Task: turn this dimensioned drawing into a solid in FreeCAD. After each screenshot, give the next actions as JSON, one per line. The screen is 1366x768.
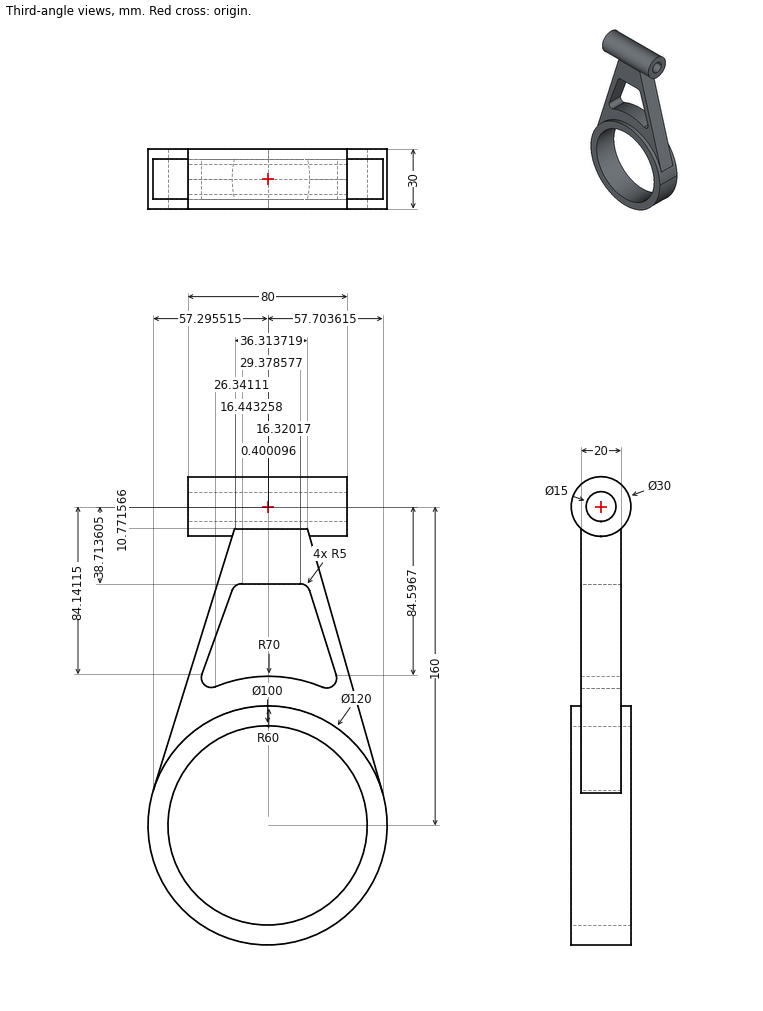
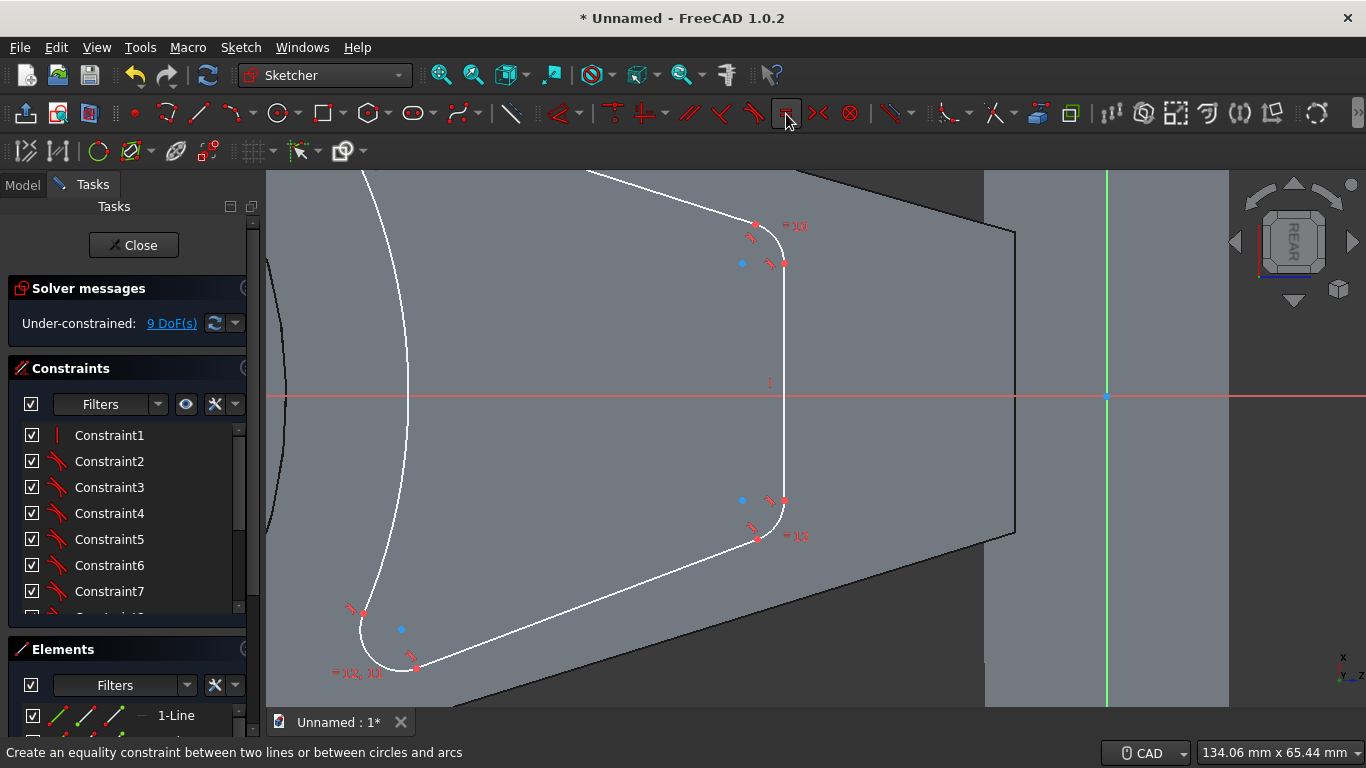
{"action": "left_click", "coordinate": [558, 114]}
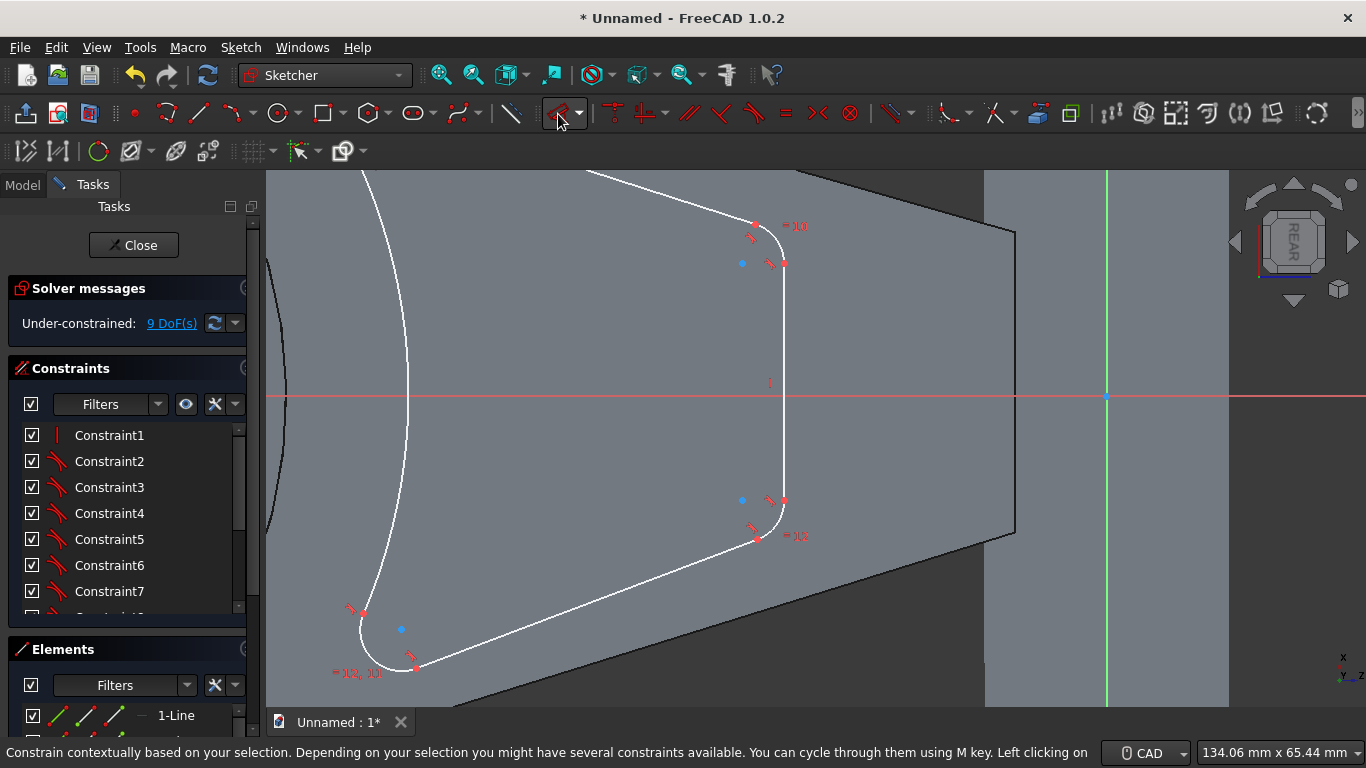
{"action": "left_click", "coordinate": [781, 248]}
{"action": "left_click", "coordinate": [811, 236]}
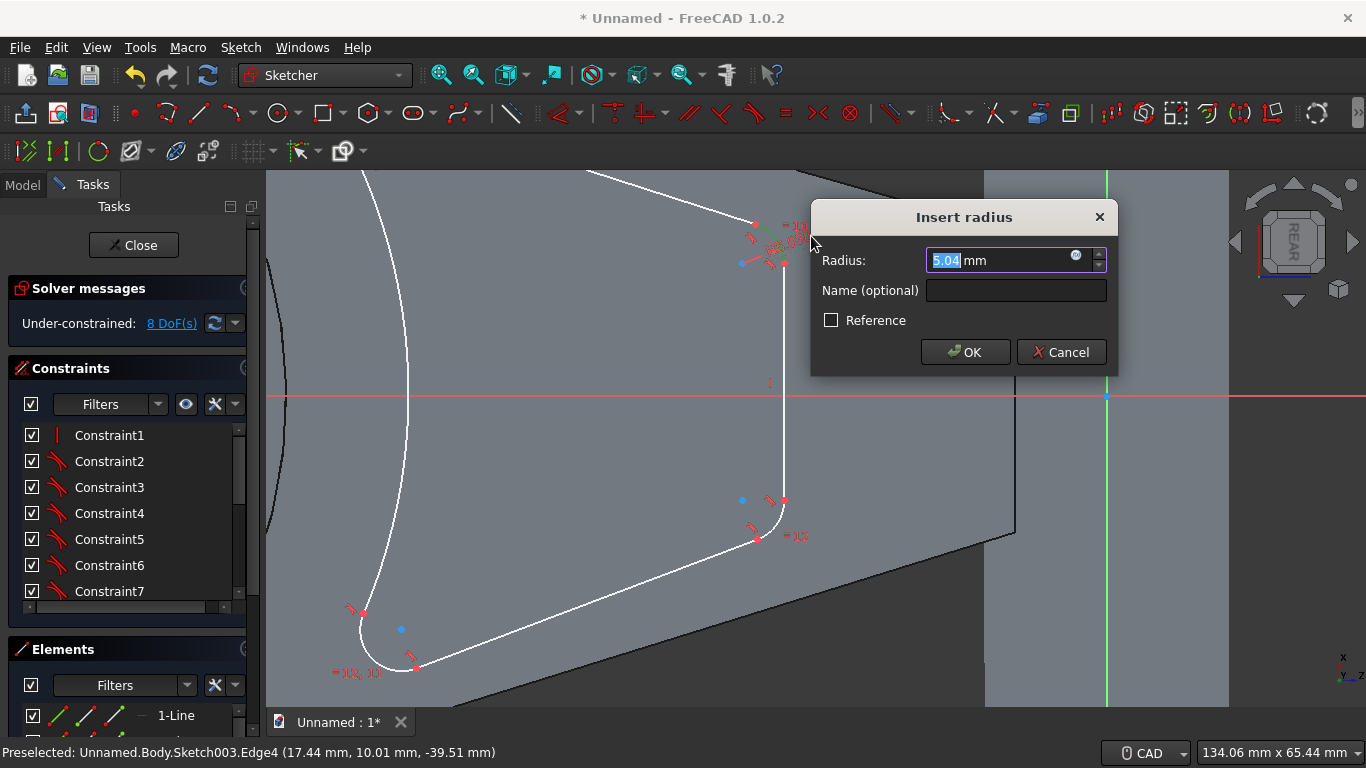
{"action": "type", "text": "5"}
{"action": "key", "text": "Return"}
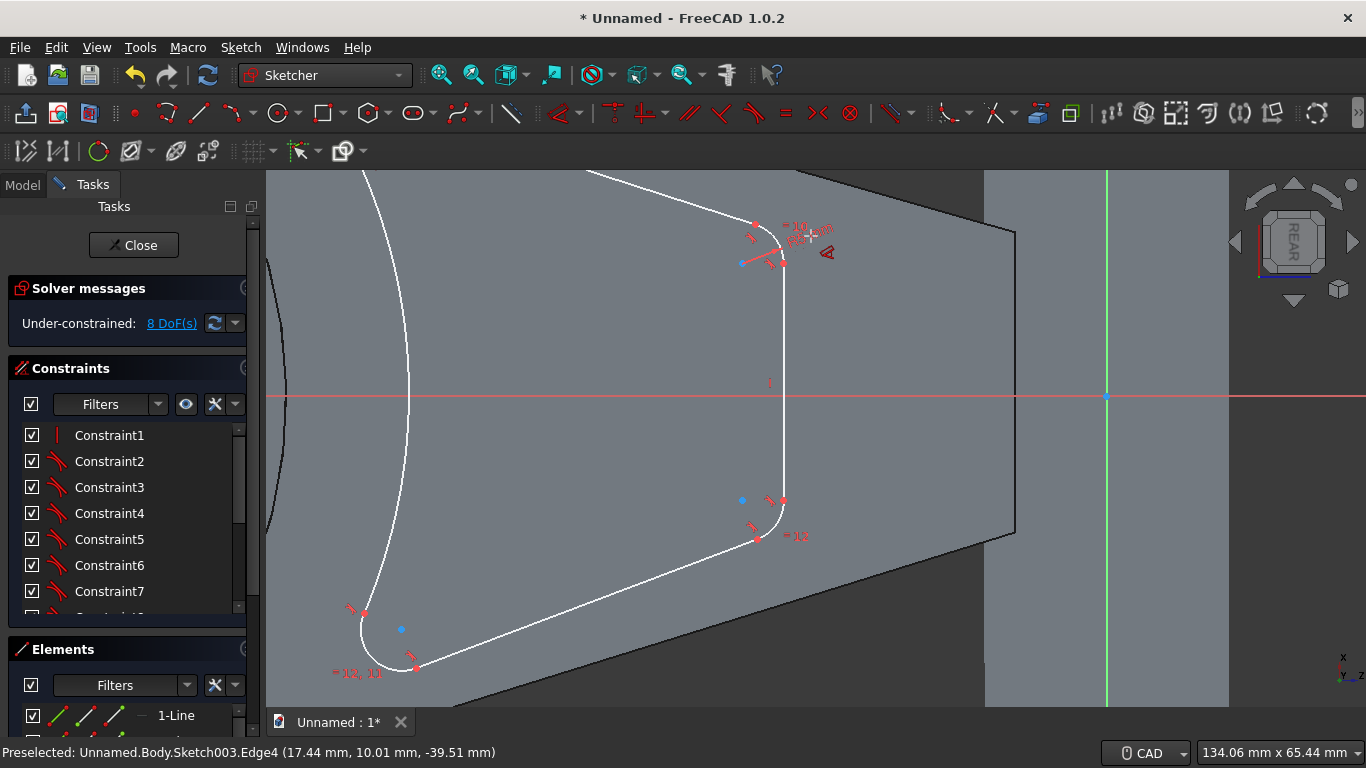
{"action": "left_click", "coordinate": [402, 482]}
{"action": "left_click", "coordinate": [434, 487]}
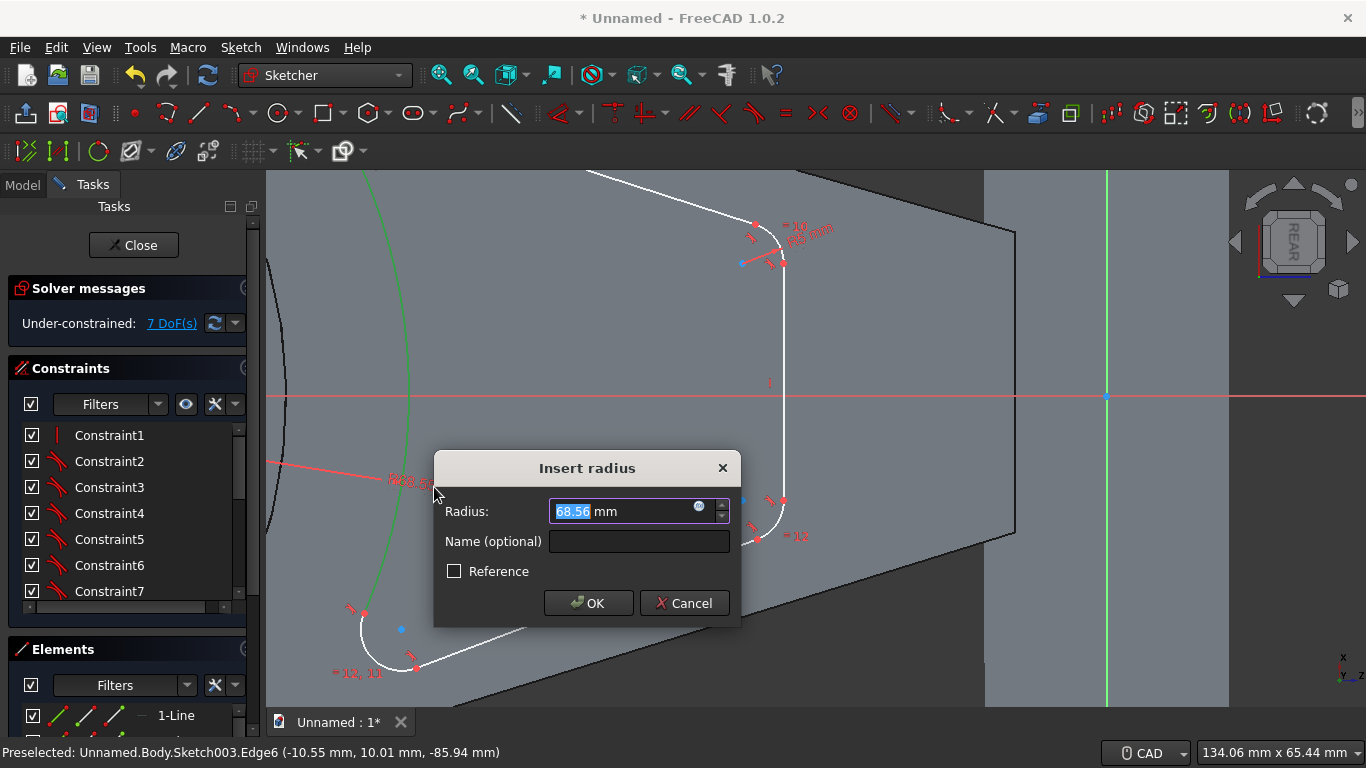
{"action": "type", "text": "70"}
{"action": "key", "text": "Return"}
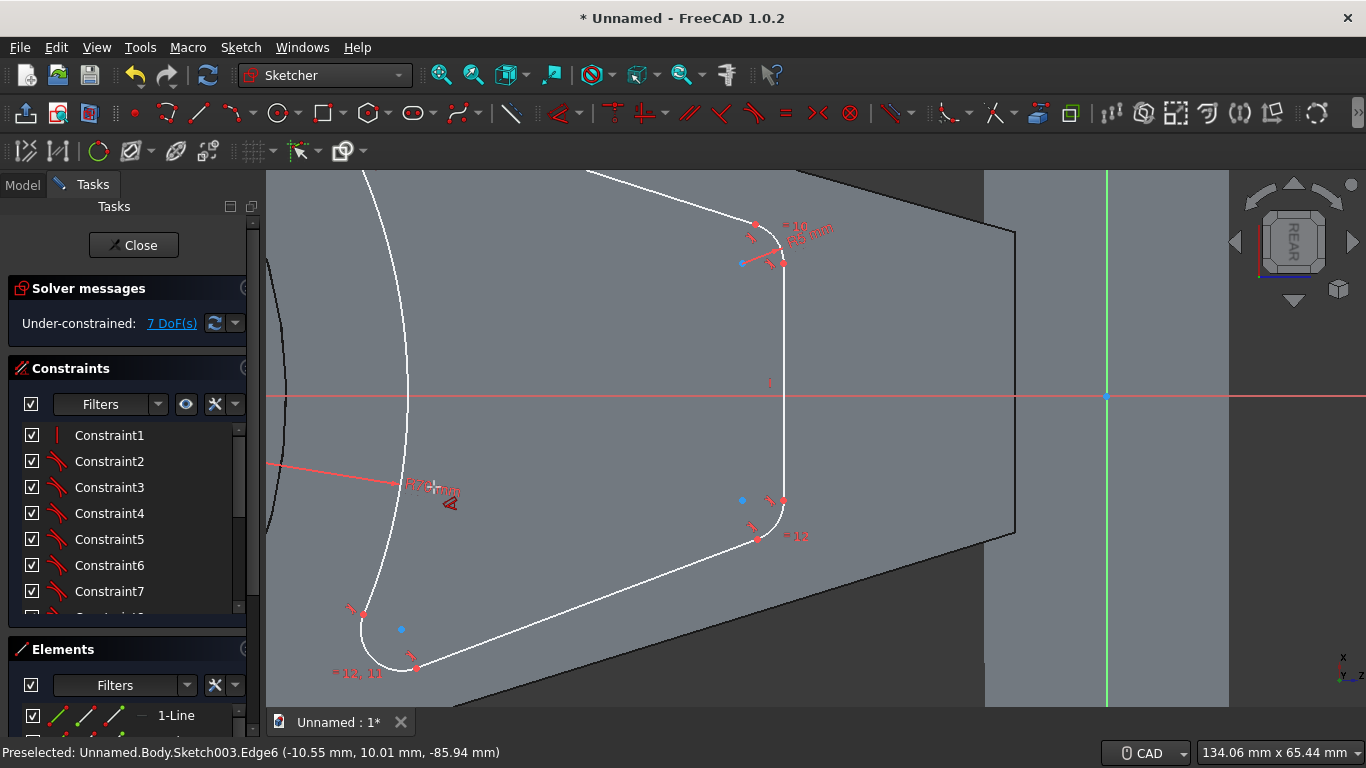
{"action": "scroll", "coordinate": [773, 537], "scroll_direction": "down", "scroll_amount": 2}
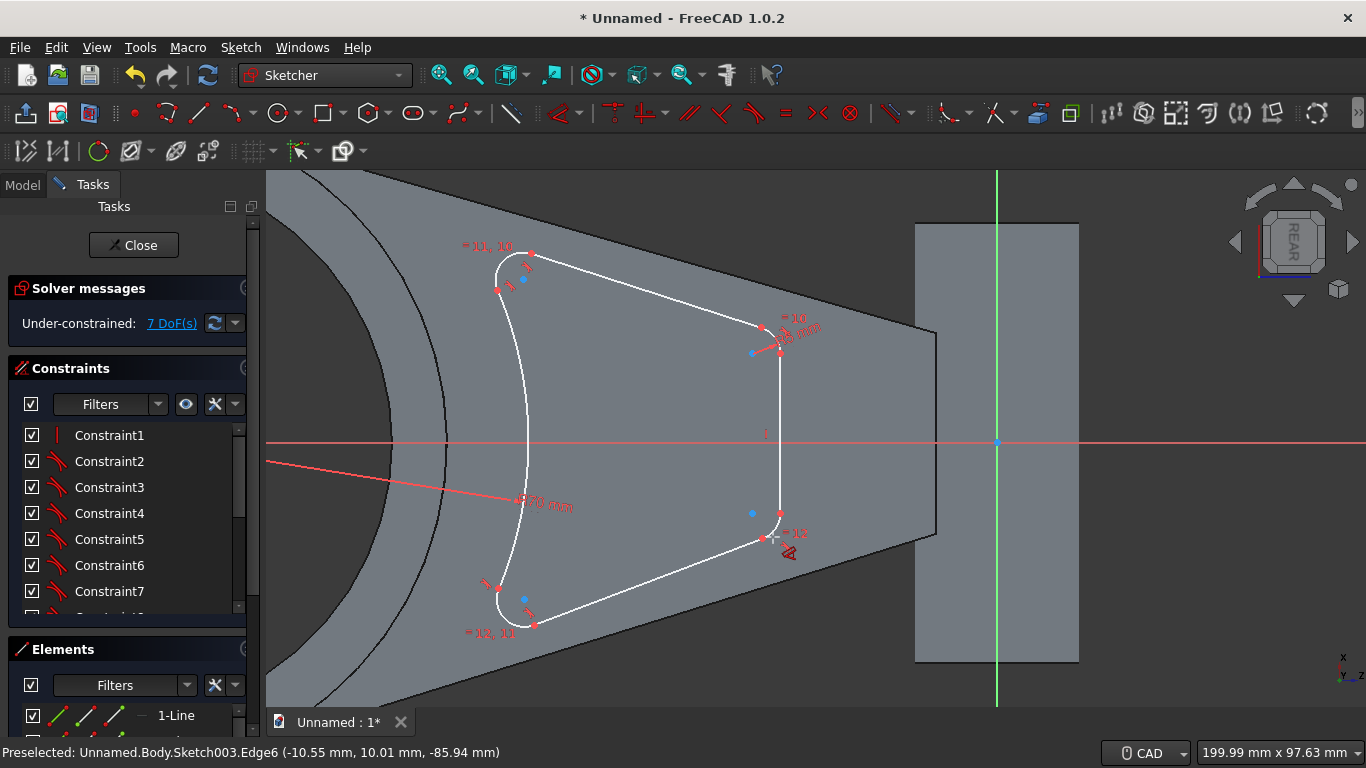
{"action": "left_click", "coordinate": [532, 254]}
{"action": "left_click", "coordinate": [764, 220]}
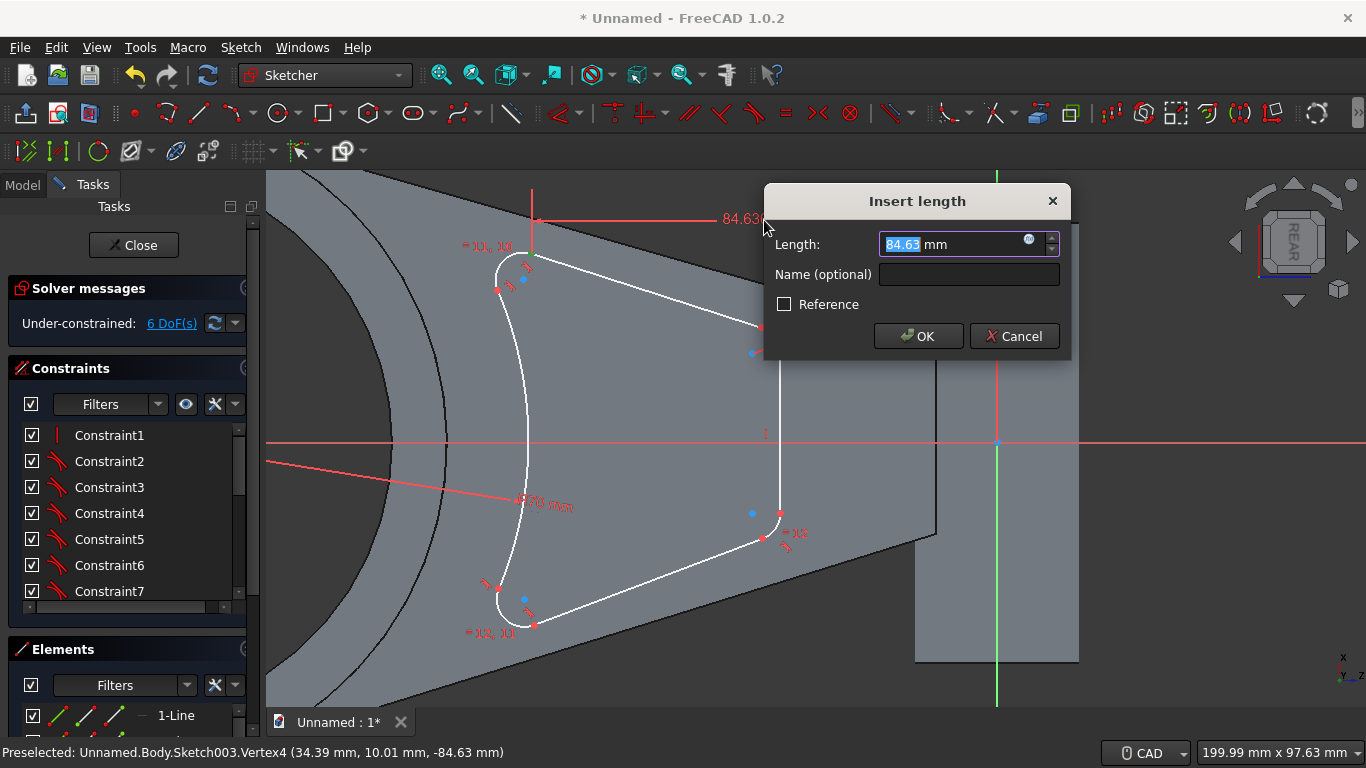
{"action": "type", "text": "84.5967"}
{"action": "key", "text": "Return"}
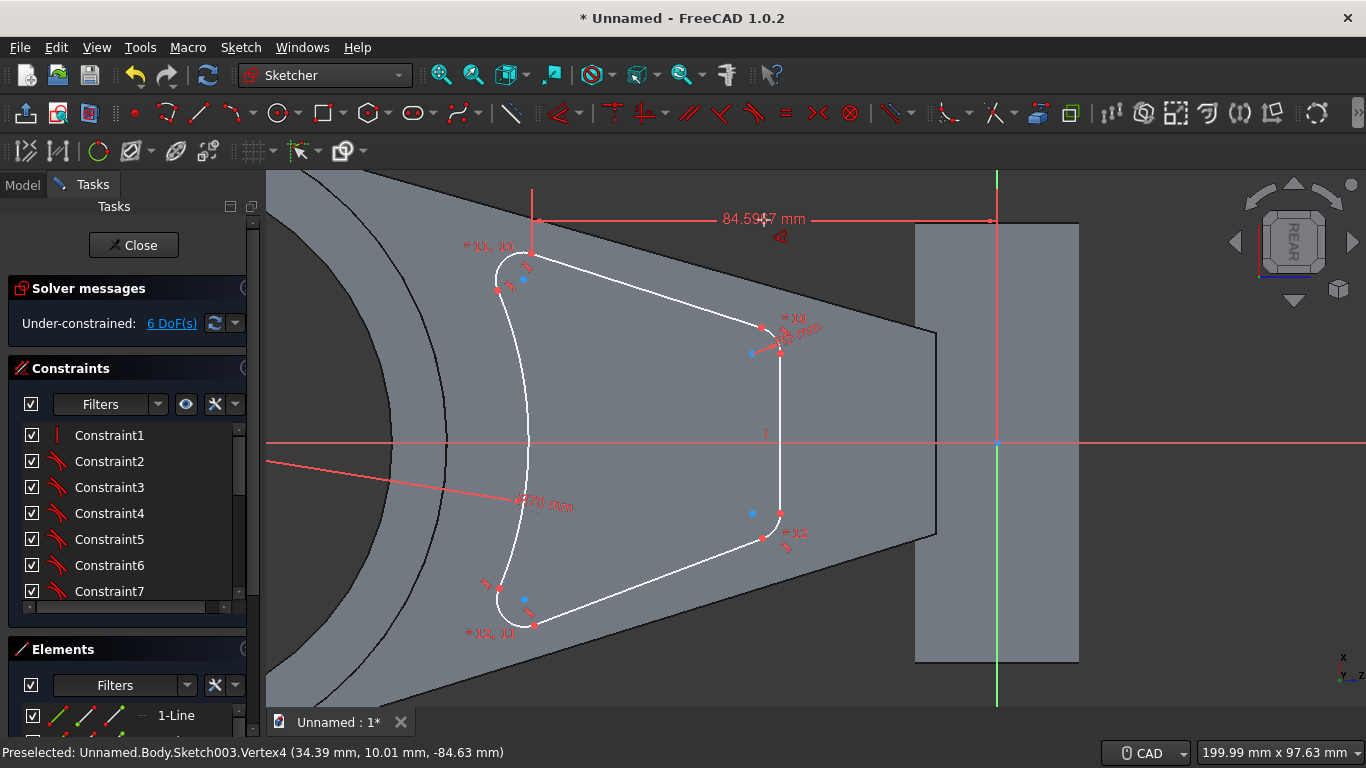
{"action": "left_click", "coordinate": [780, 465]}
{"action": "left_click", "coordinate": [814, 397]}